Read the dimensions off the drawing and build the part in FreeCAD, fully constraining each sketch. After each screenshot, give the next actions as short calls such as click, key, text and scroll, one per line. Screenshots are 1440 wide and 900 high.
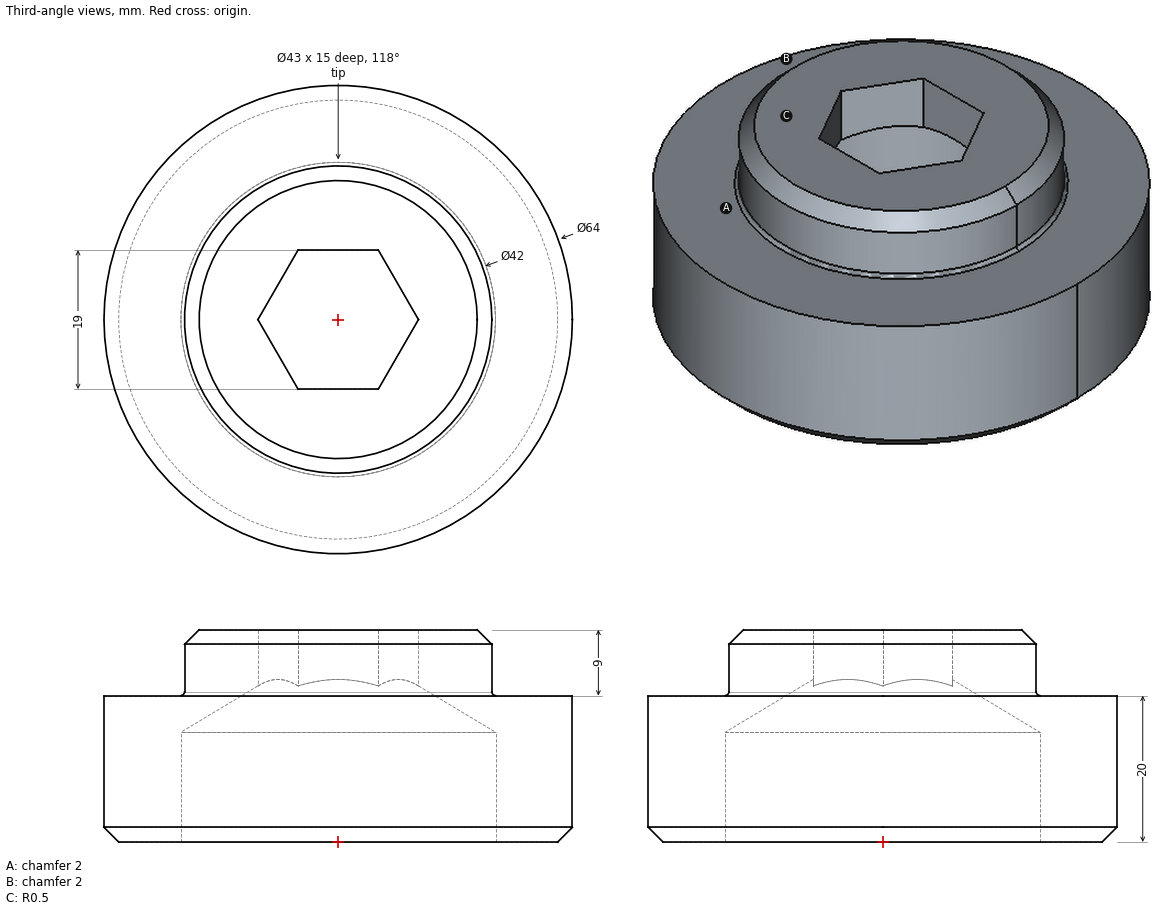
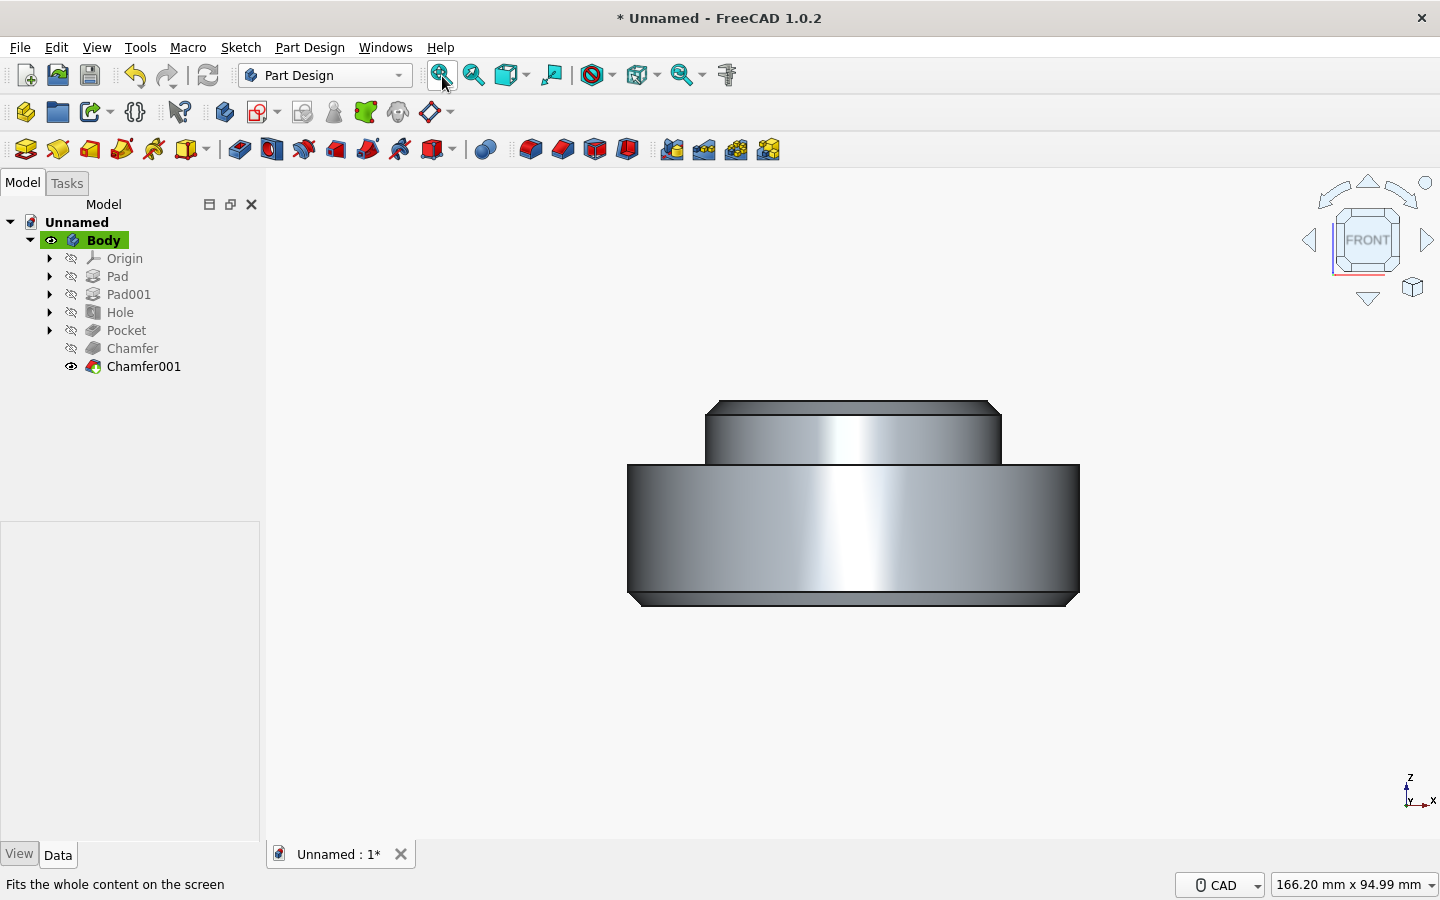
key(3)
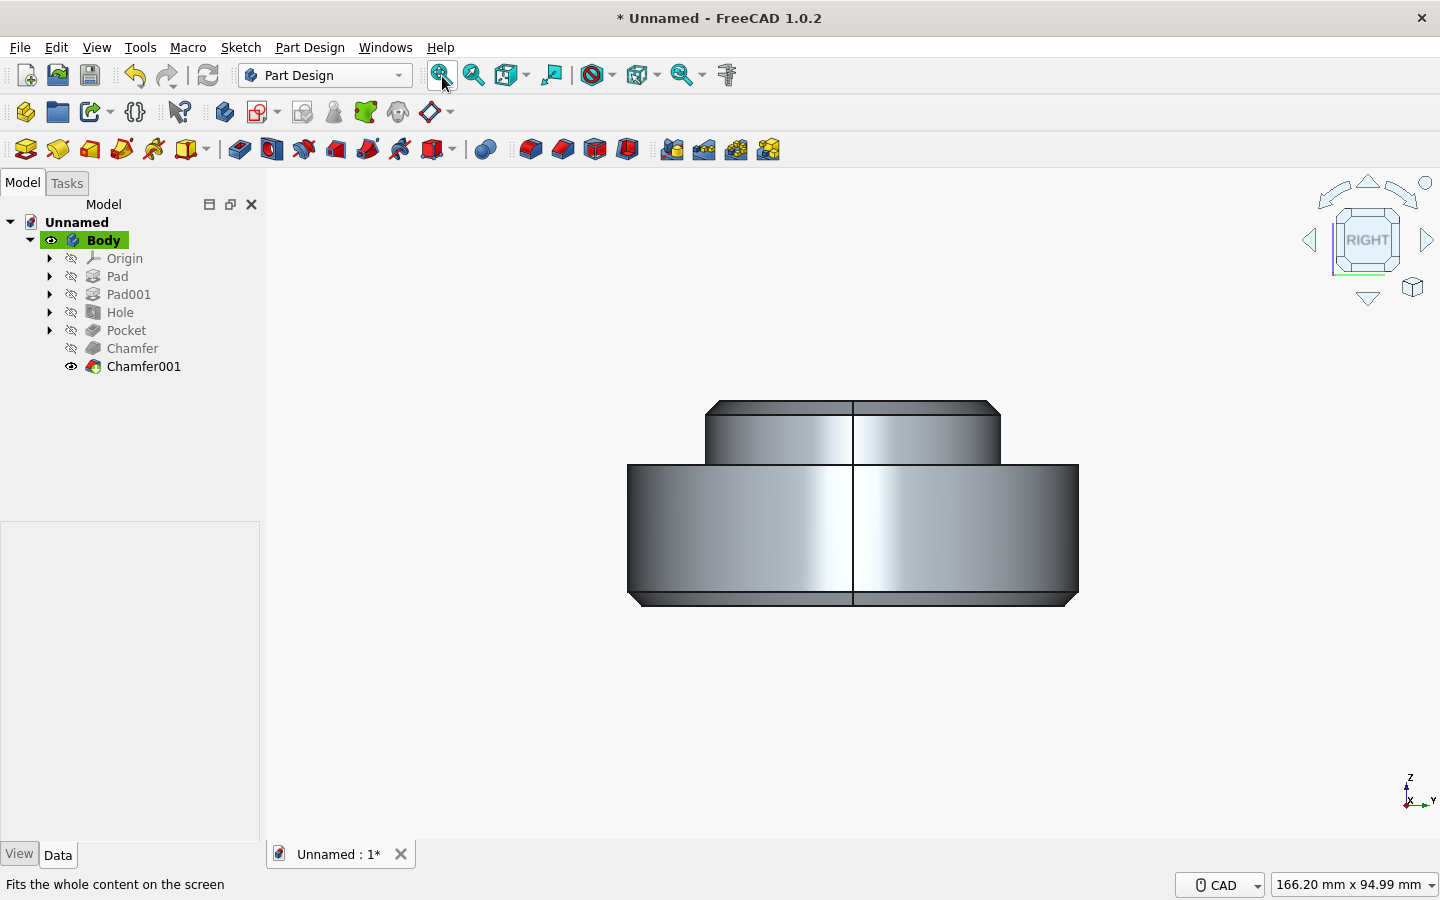
click(442, 76)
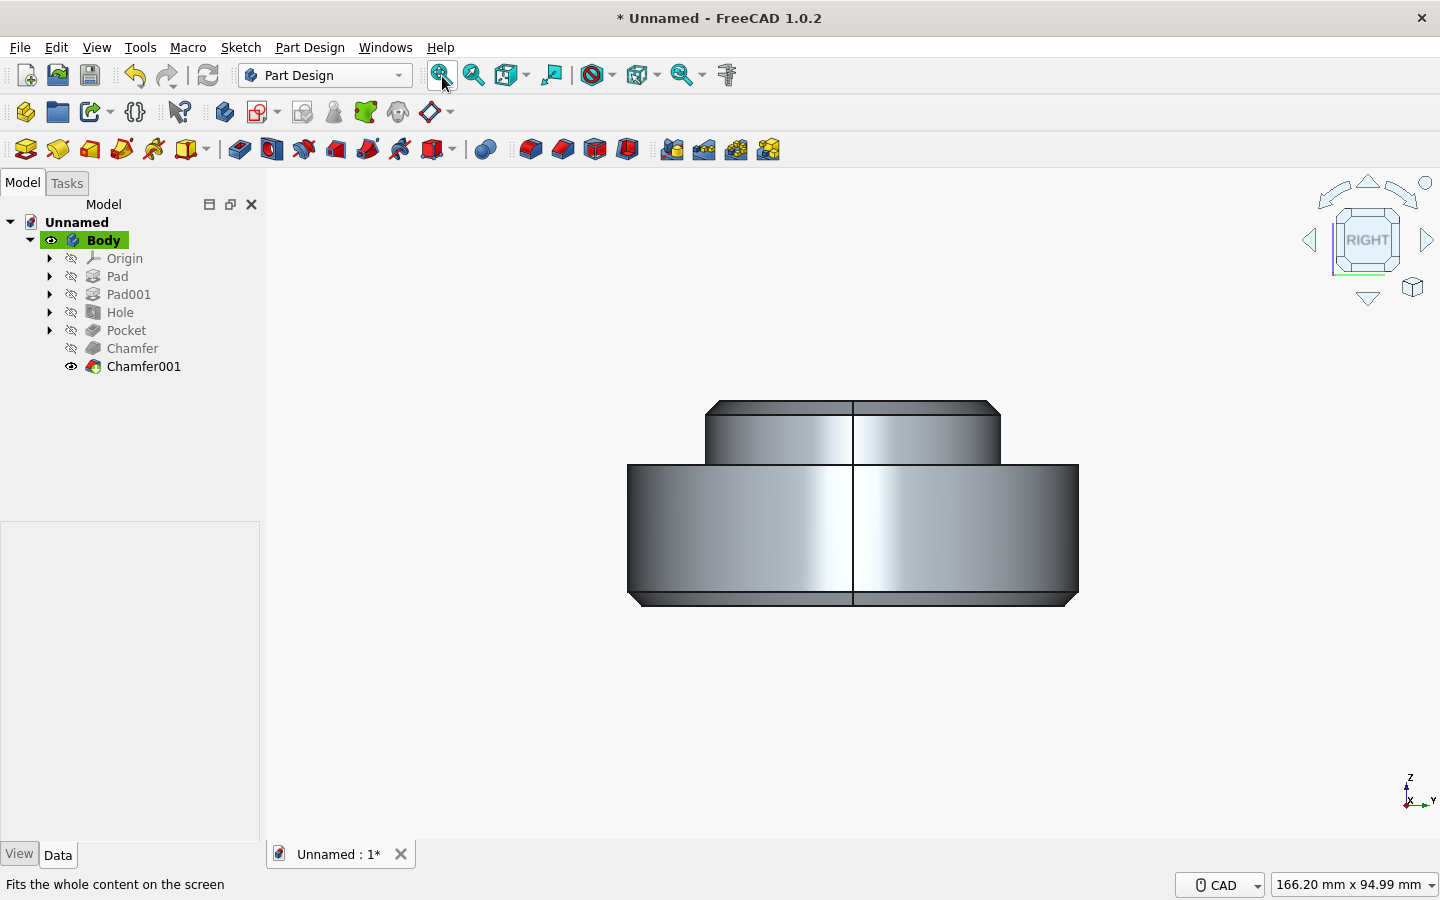
key(5)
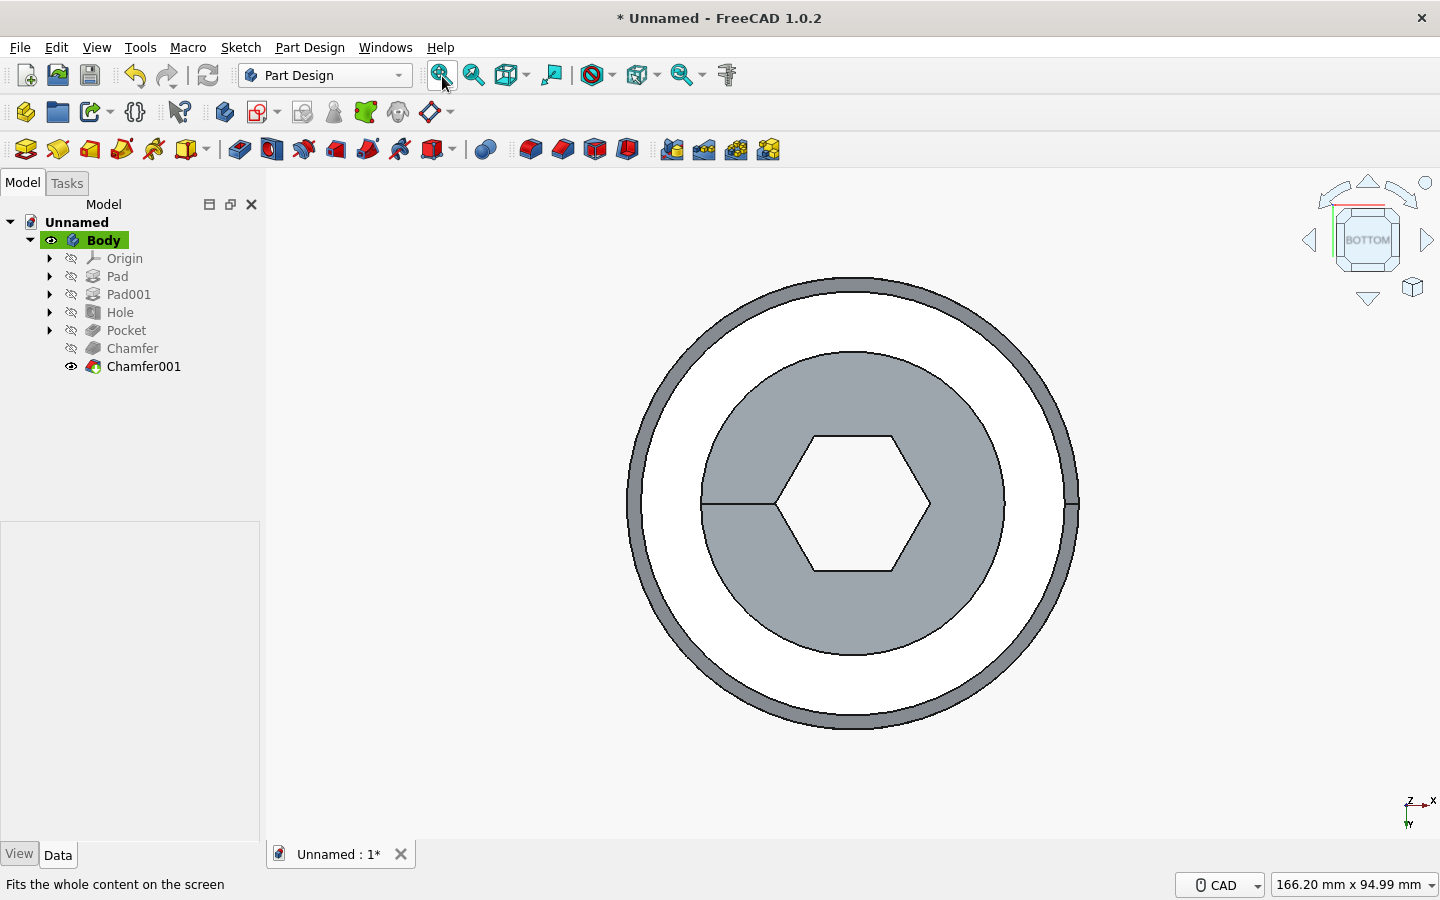
key(4)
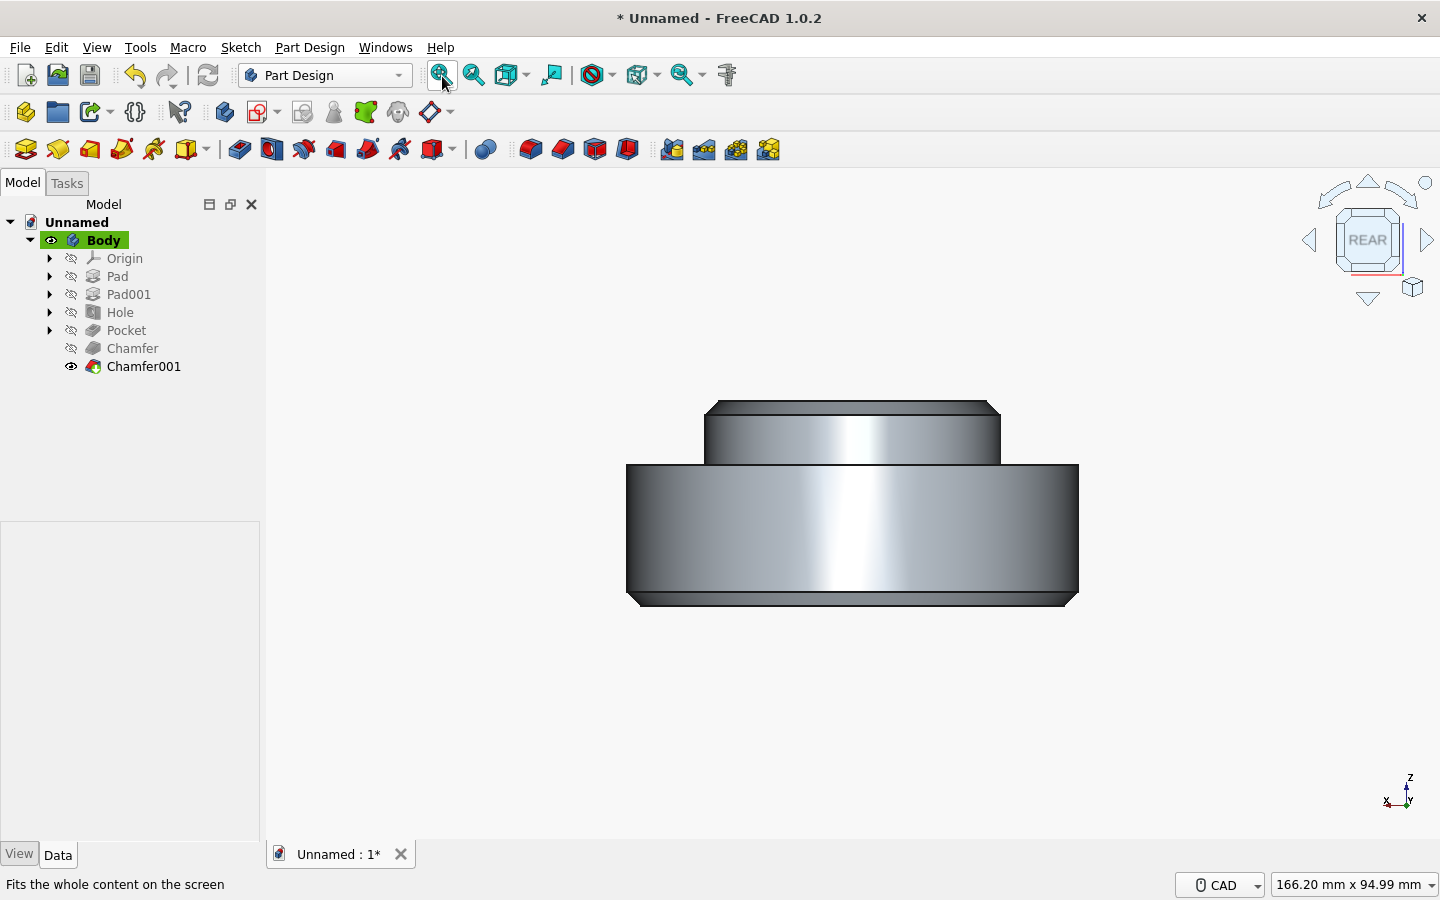
click(442, 76)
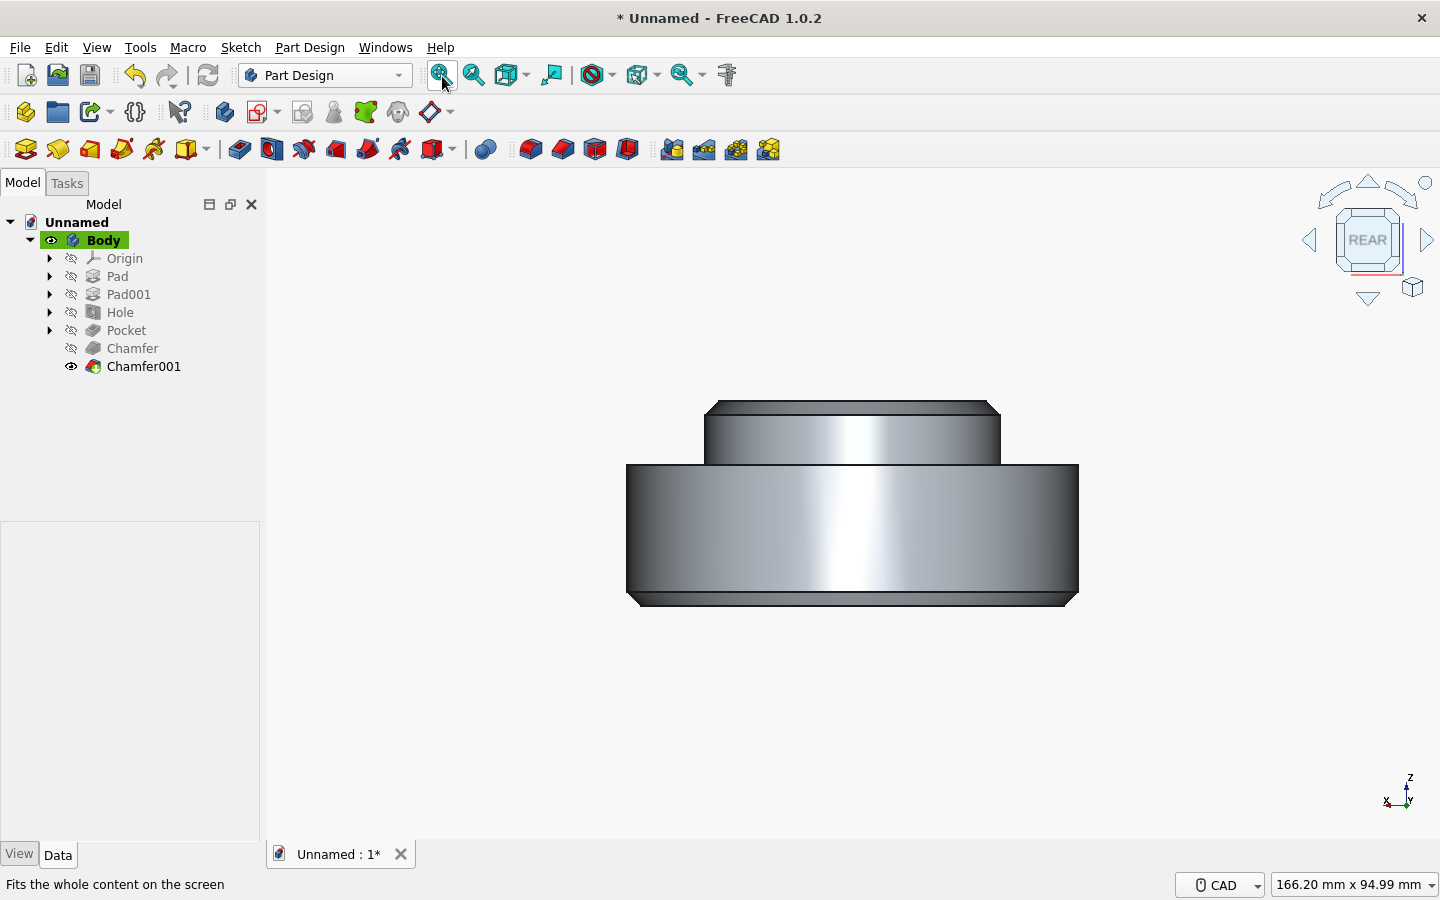
key(6)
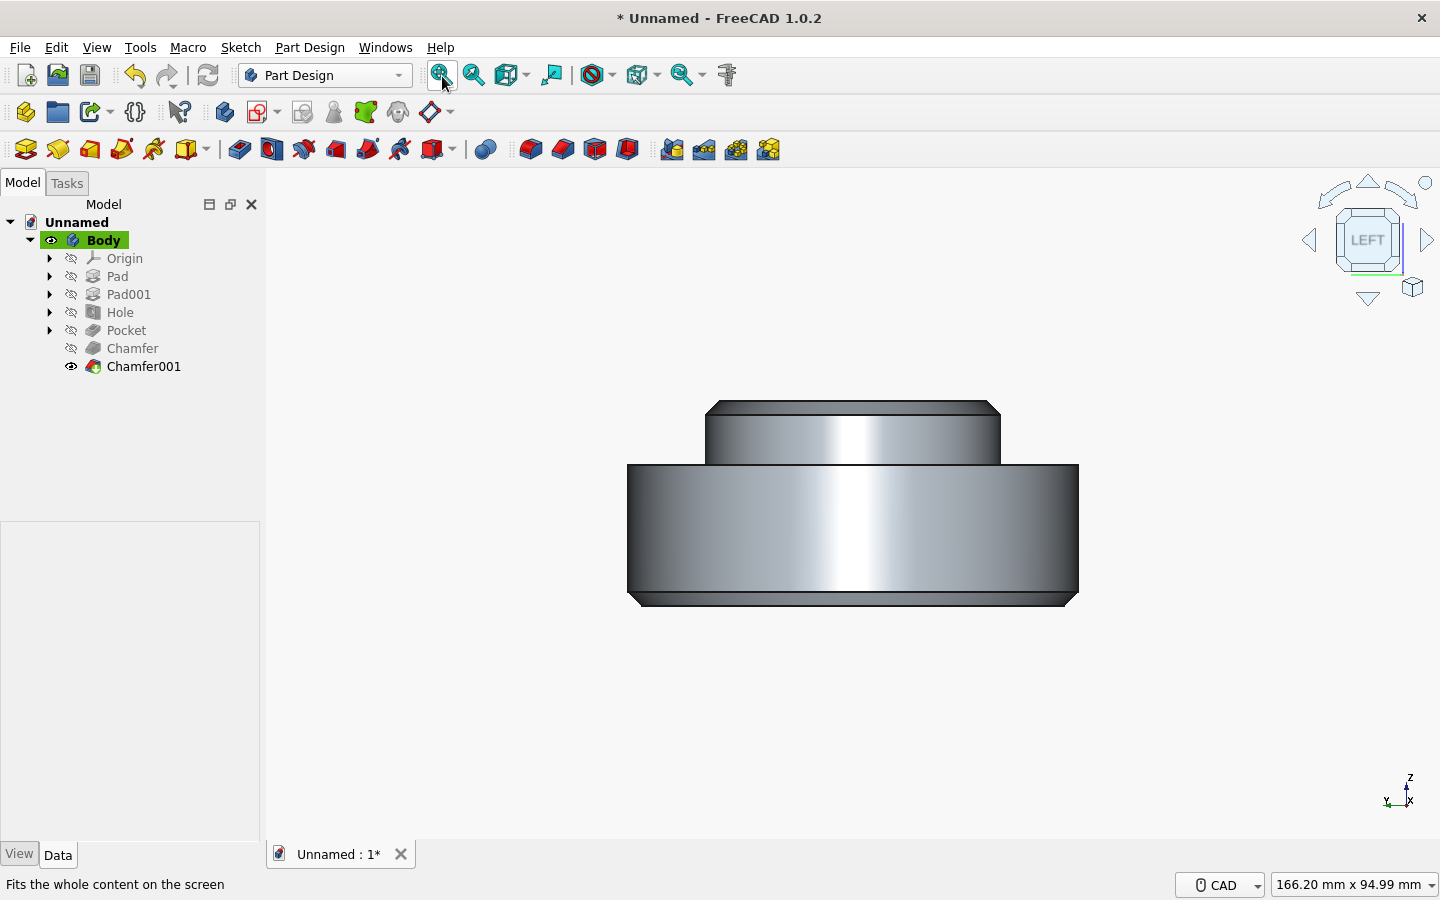
click(442, 76)